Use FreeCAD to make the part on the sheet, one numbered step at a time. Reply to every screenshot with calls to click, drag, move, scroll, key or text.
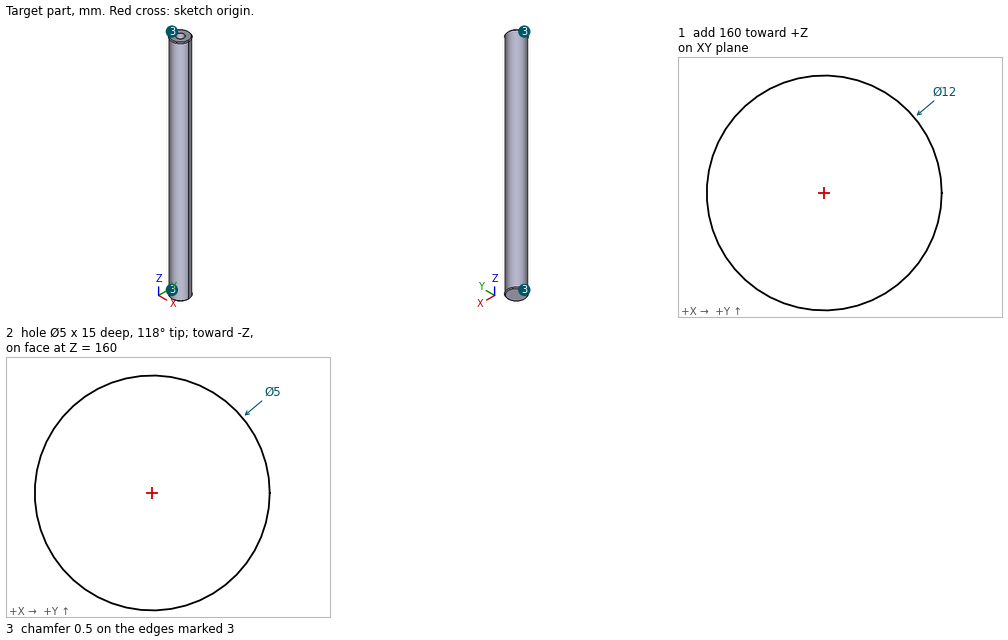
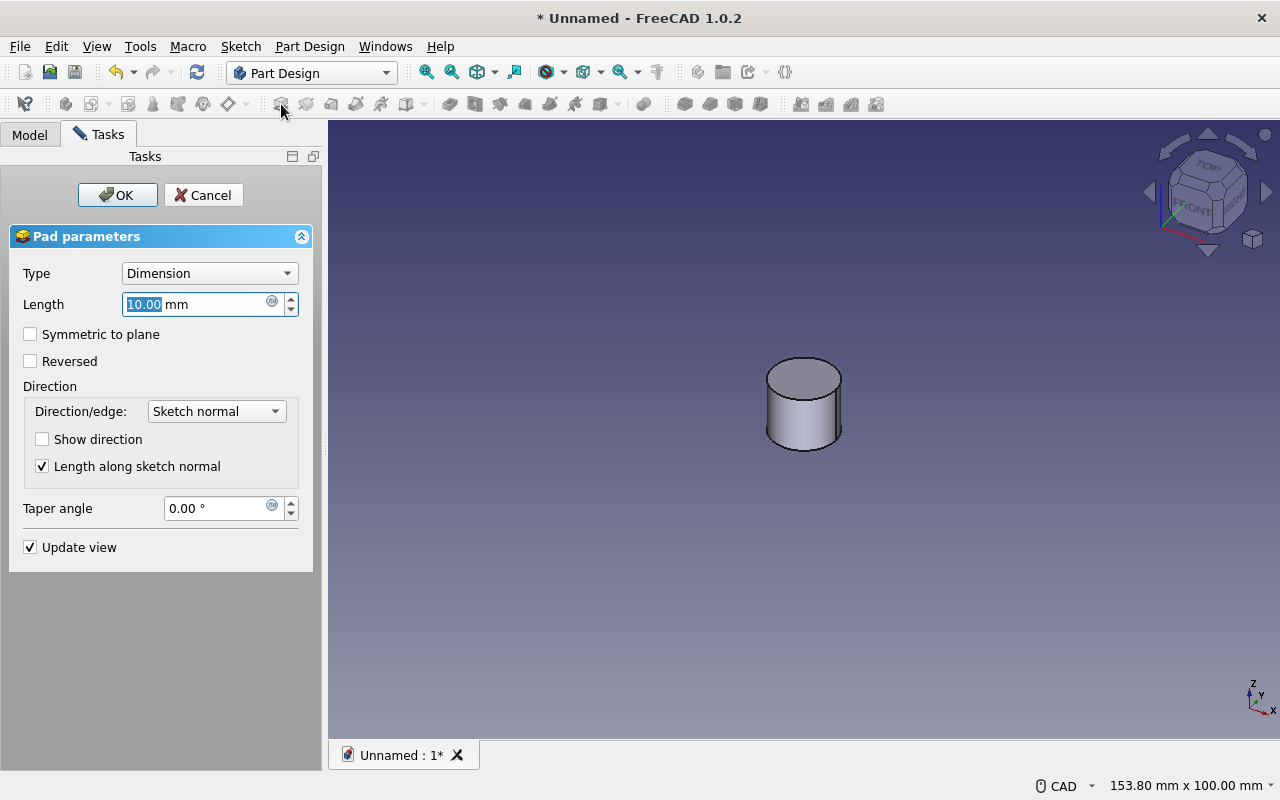
text(160)
key(Tab)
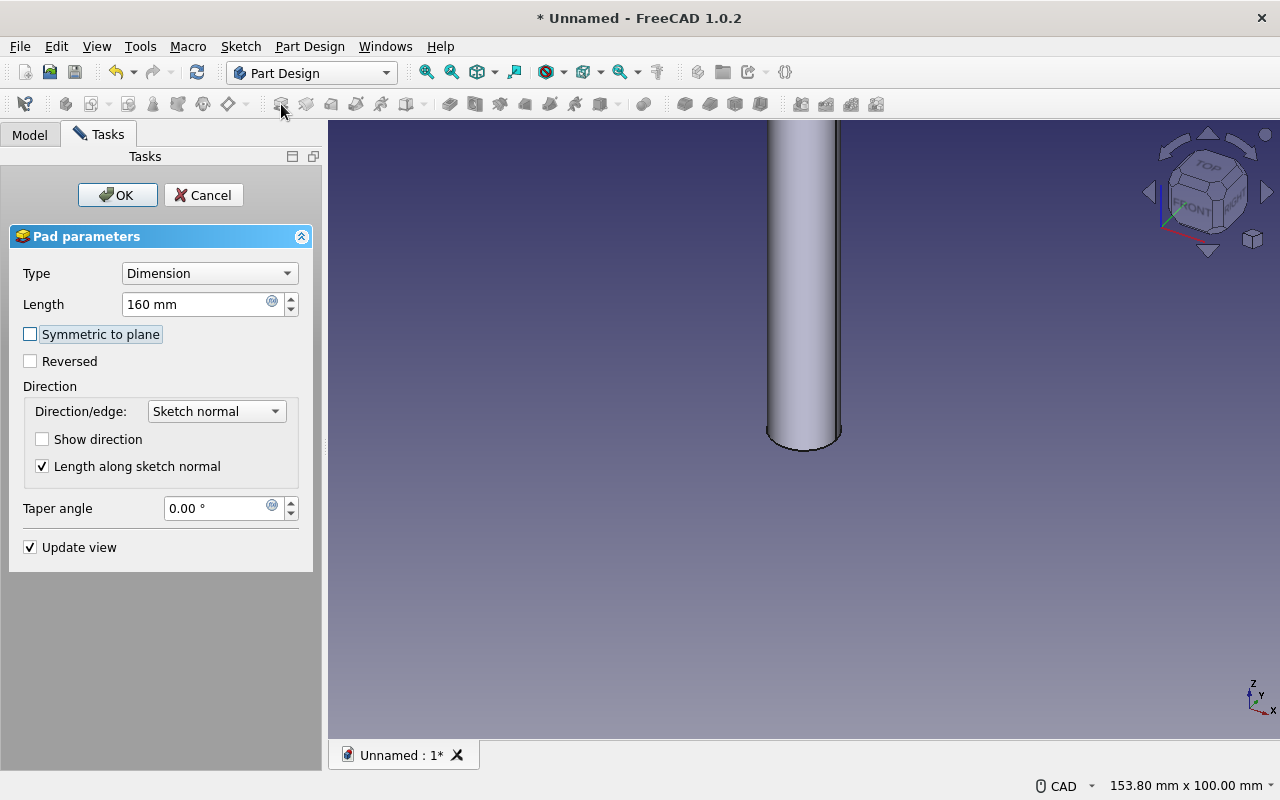
click(118, 195)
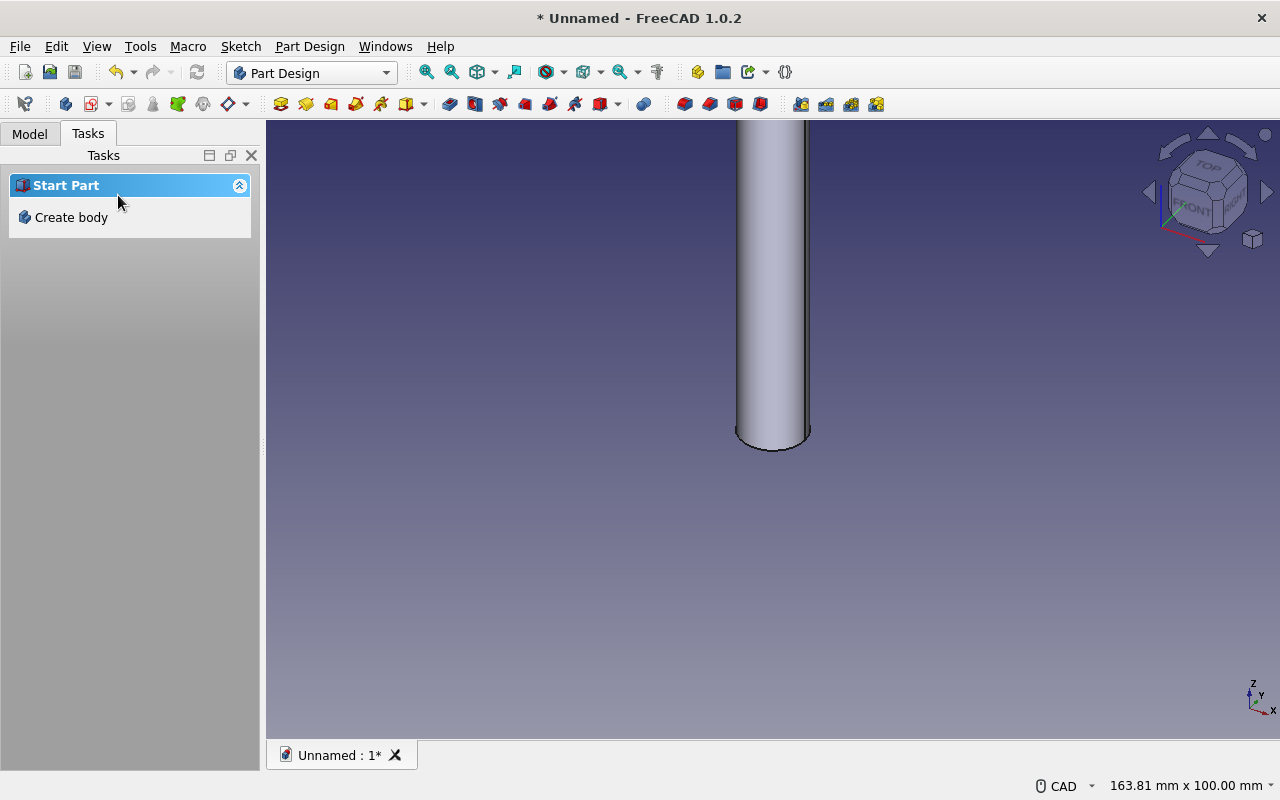
key(v)
key(f)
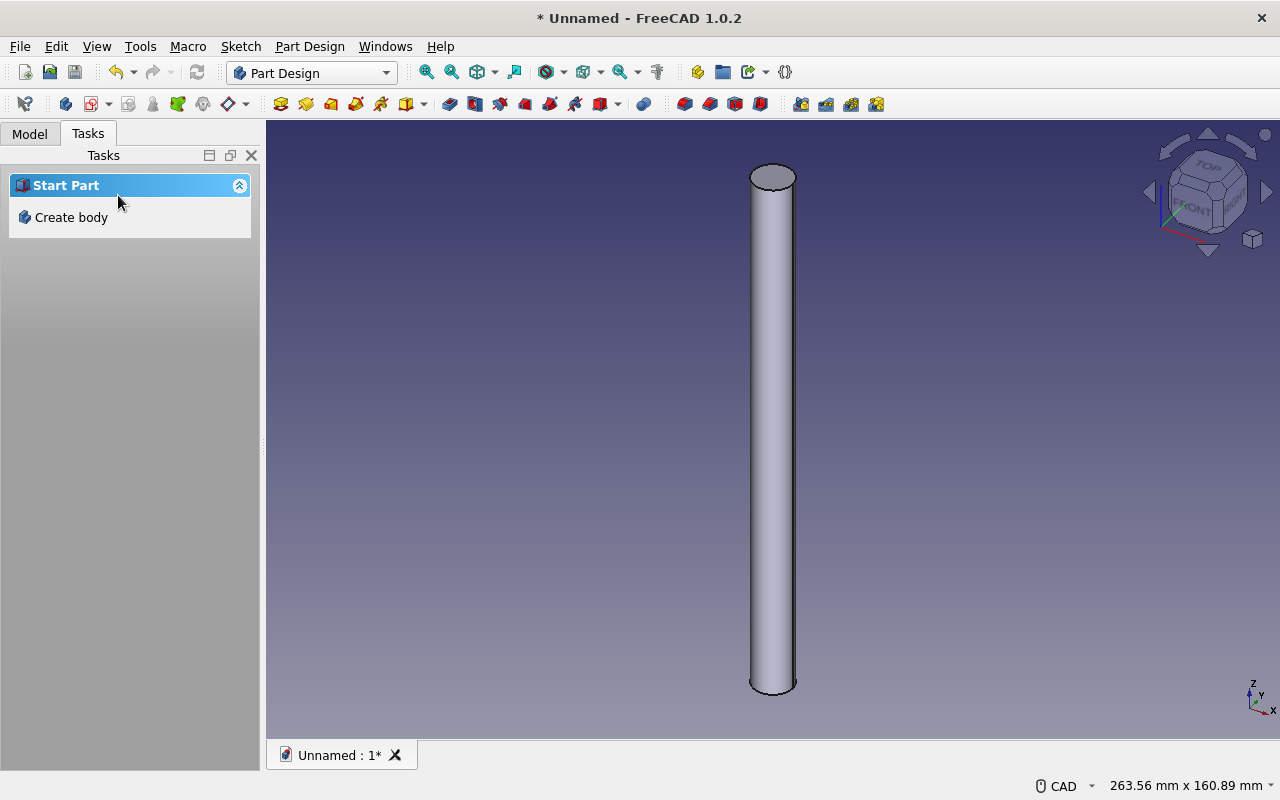
click(773, 176)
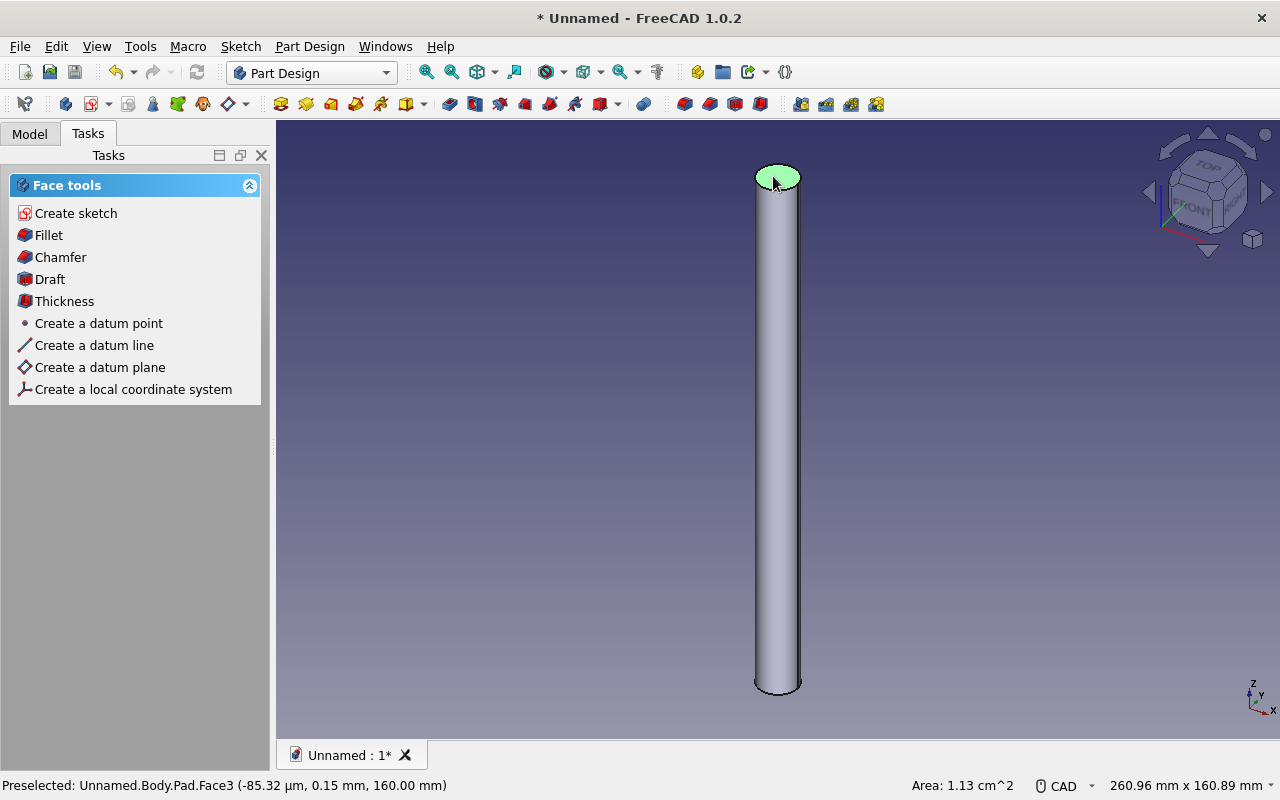
click(90, 104)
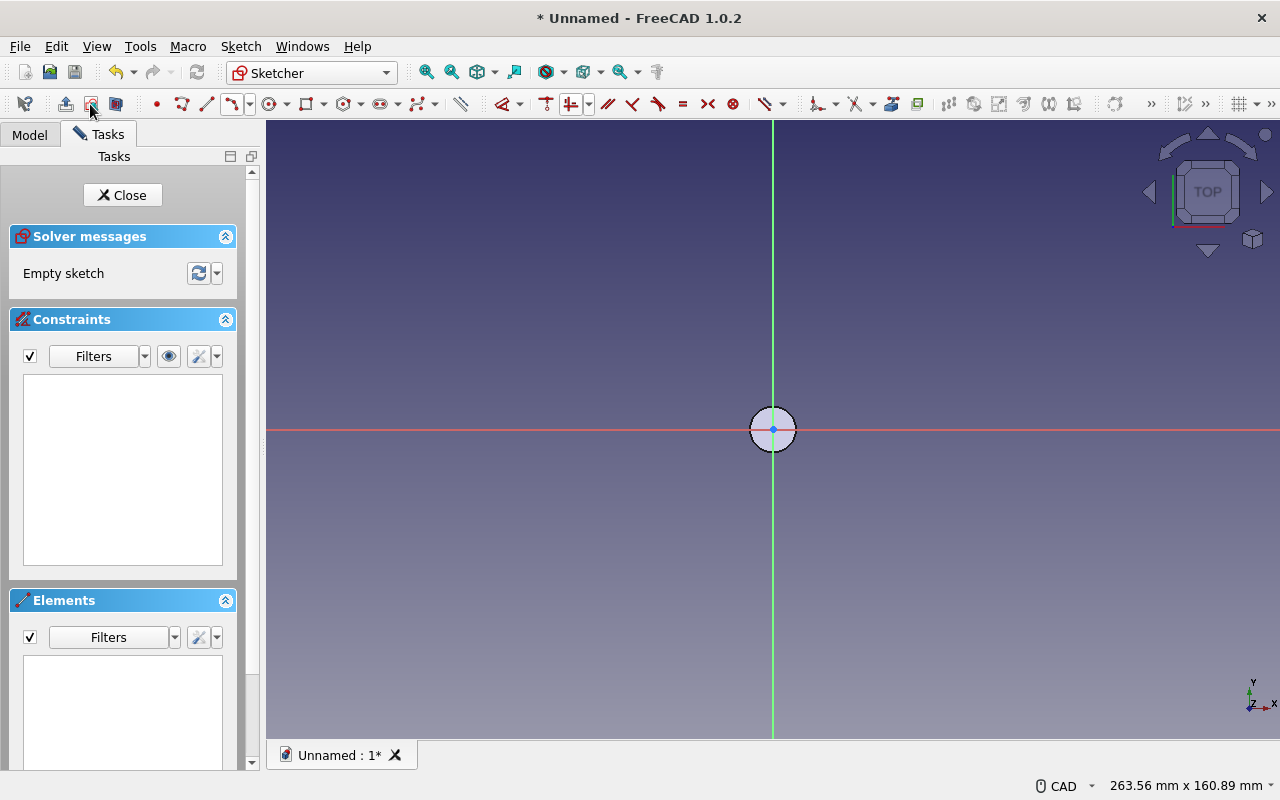
scroll(777, 430, up, 15)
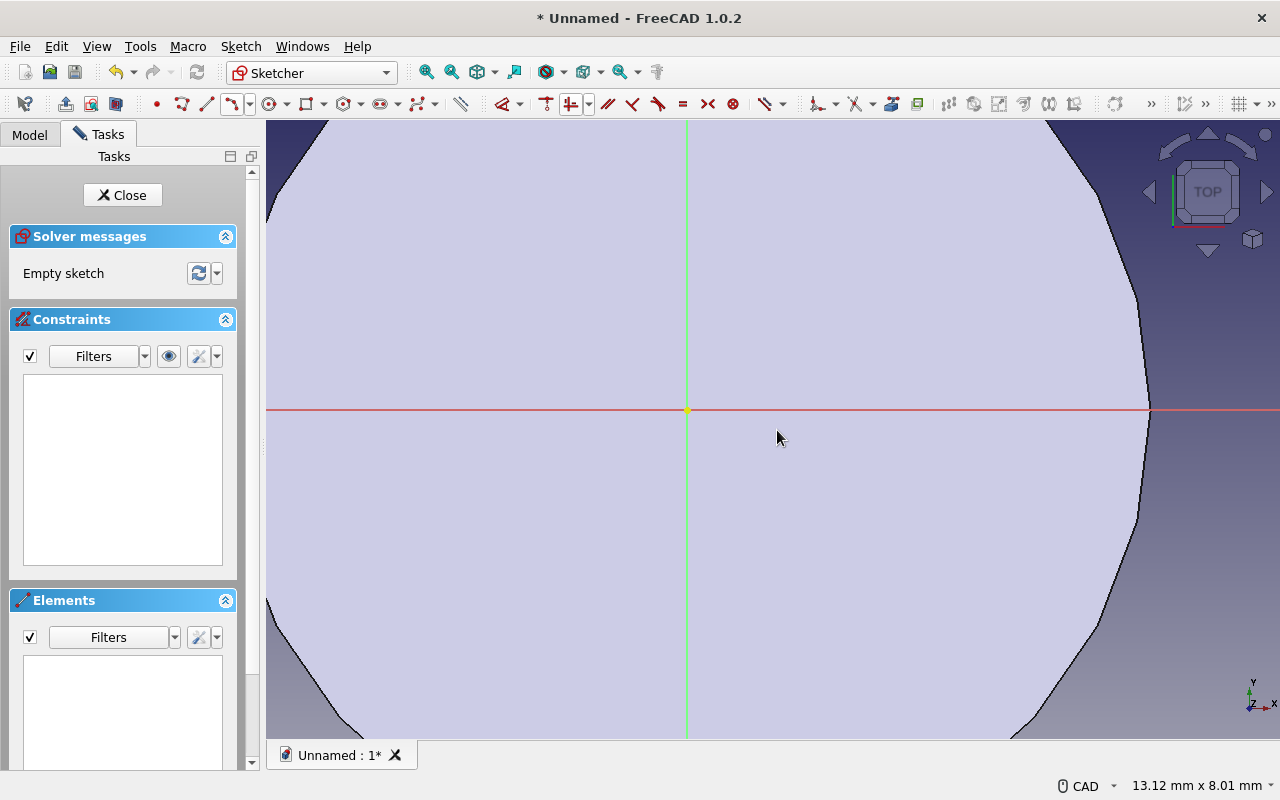
click(268, 104)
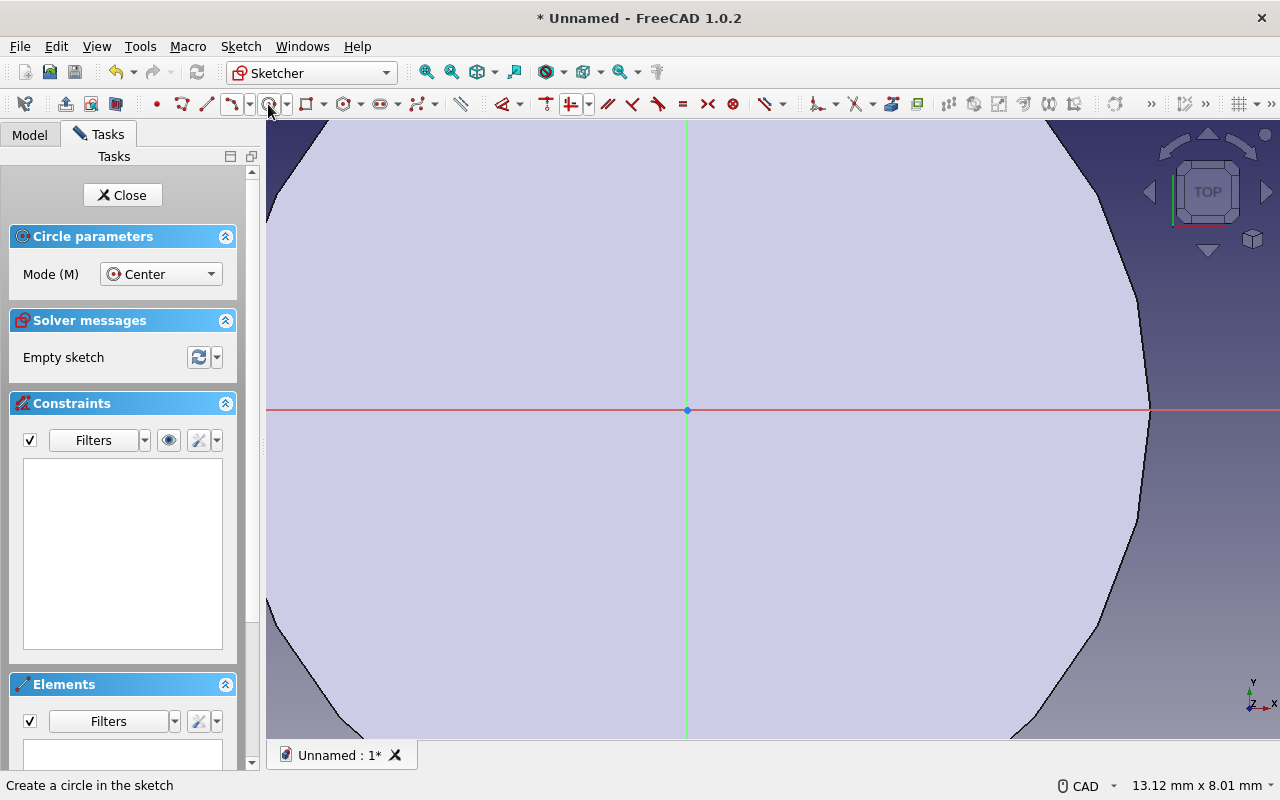
click(687, 410)
move(824, 274)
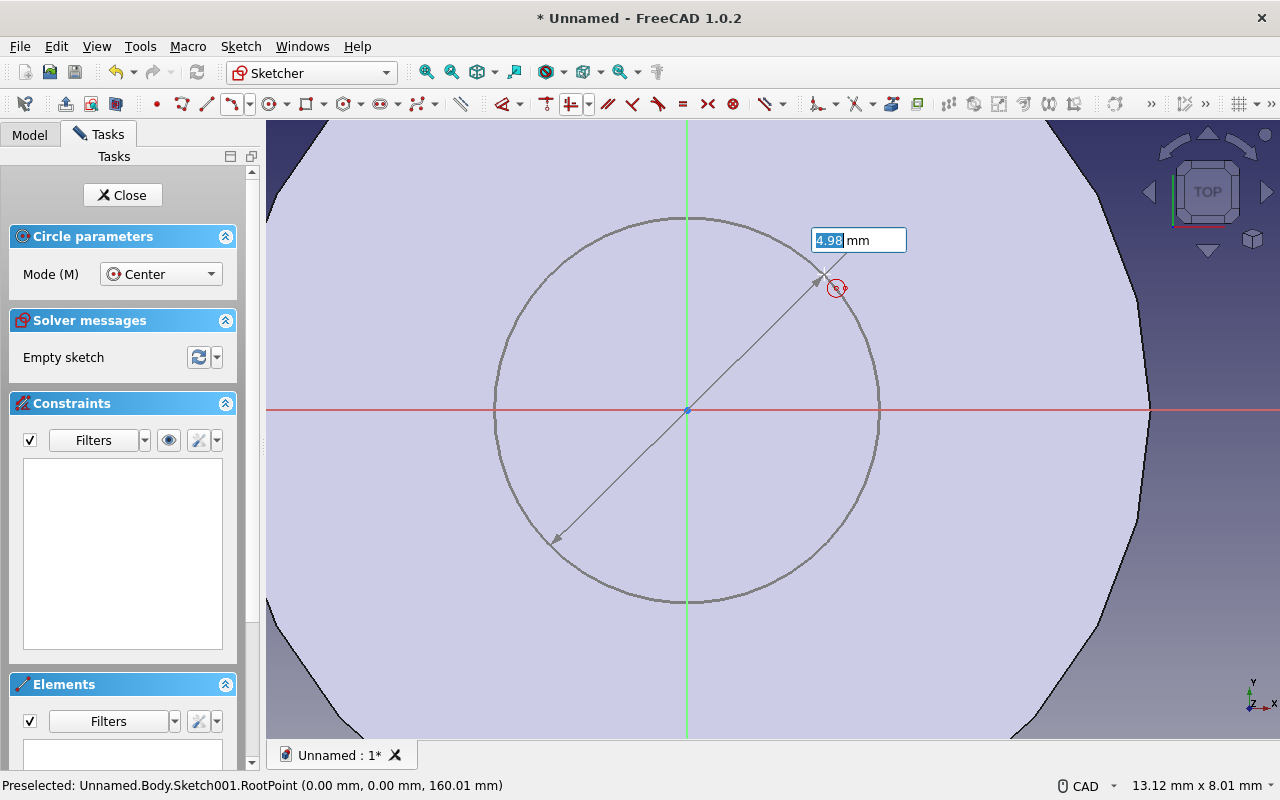
text(5)
key(Return)
key(Escape)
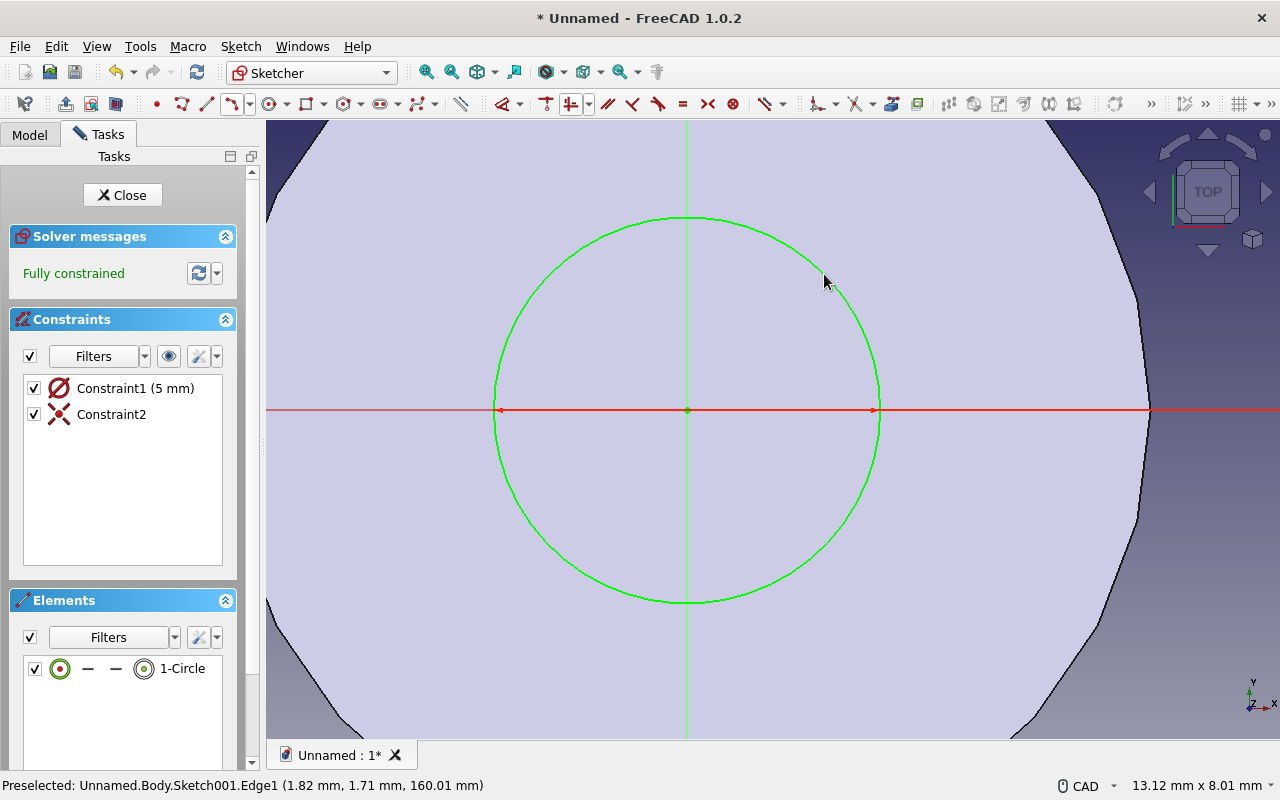
click(123, 195)